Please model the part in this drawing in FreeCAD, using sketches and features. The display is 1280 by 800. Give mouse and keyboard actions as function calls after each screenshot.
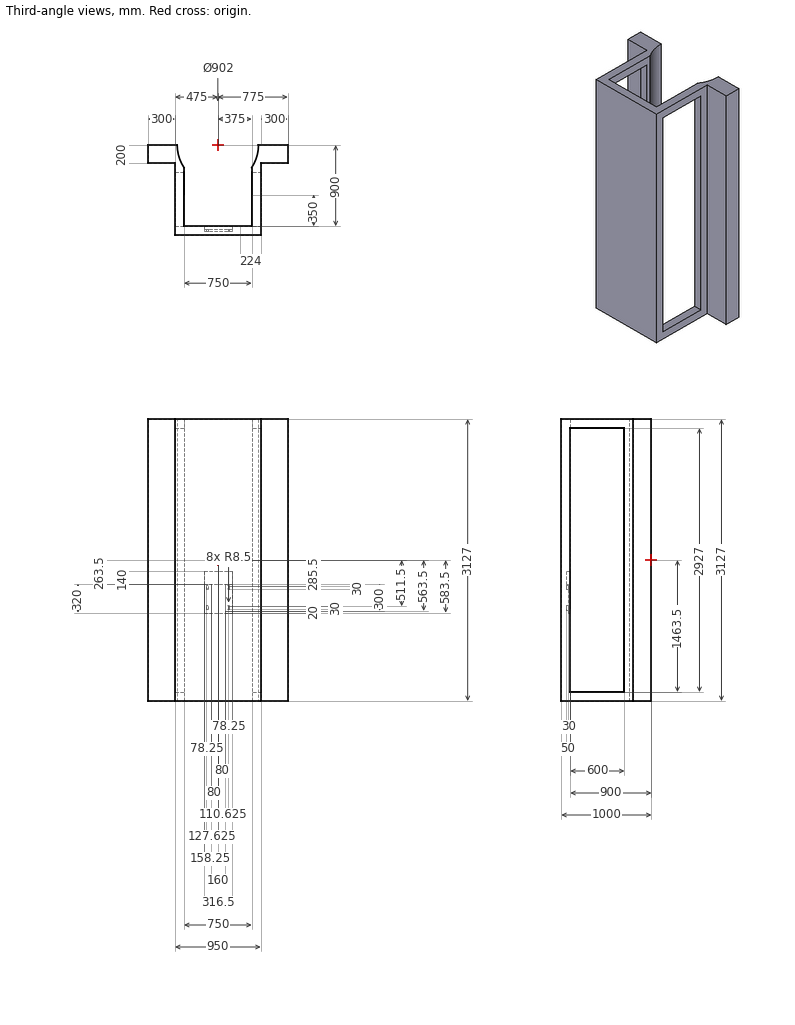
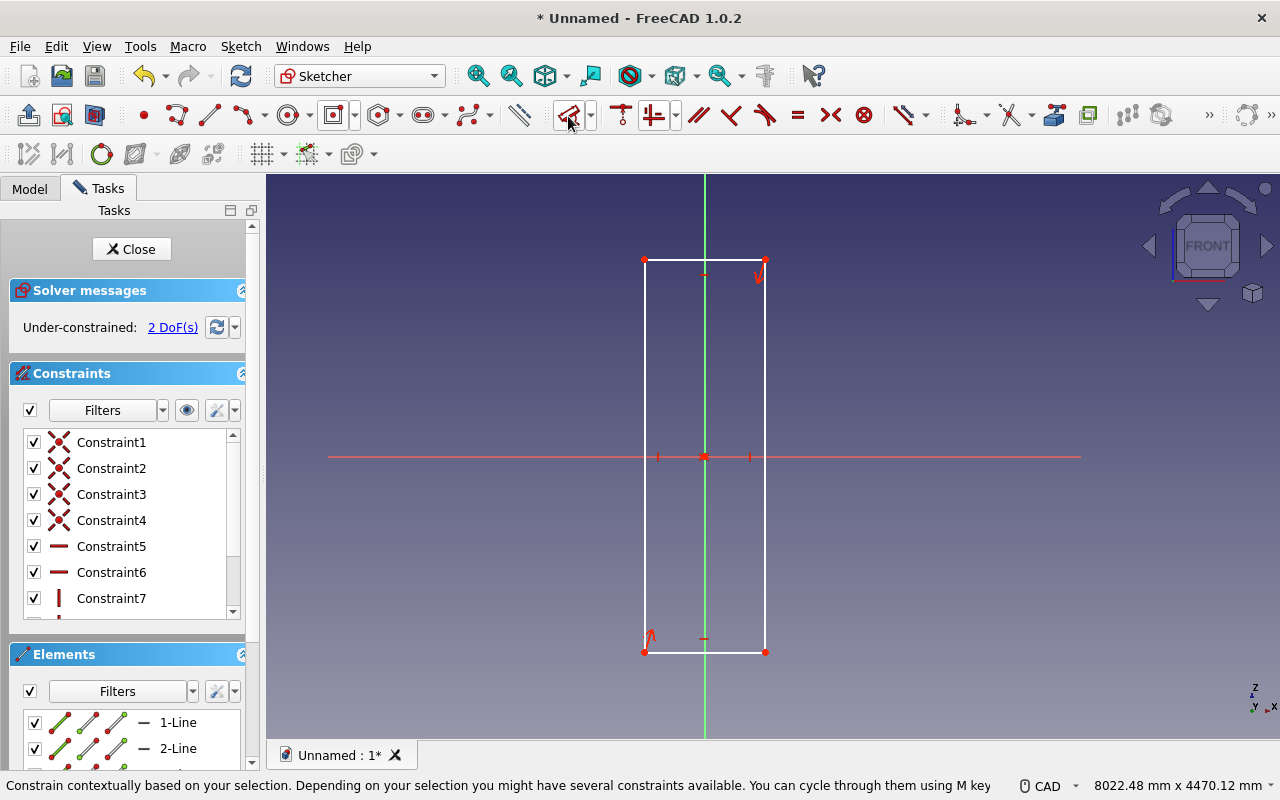
click(681, 653)
click(677, 687)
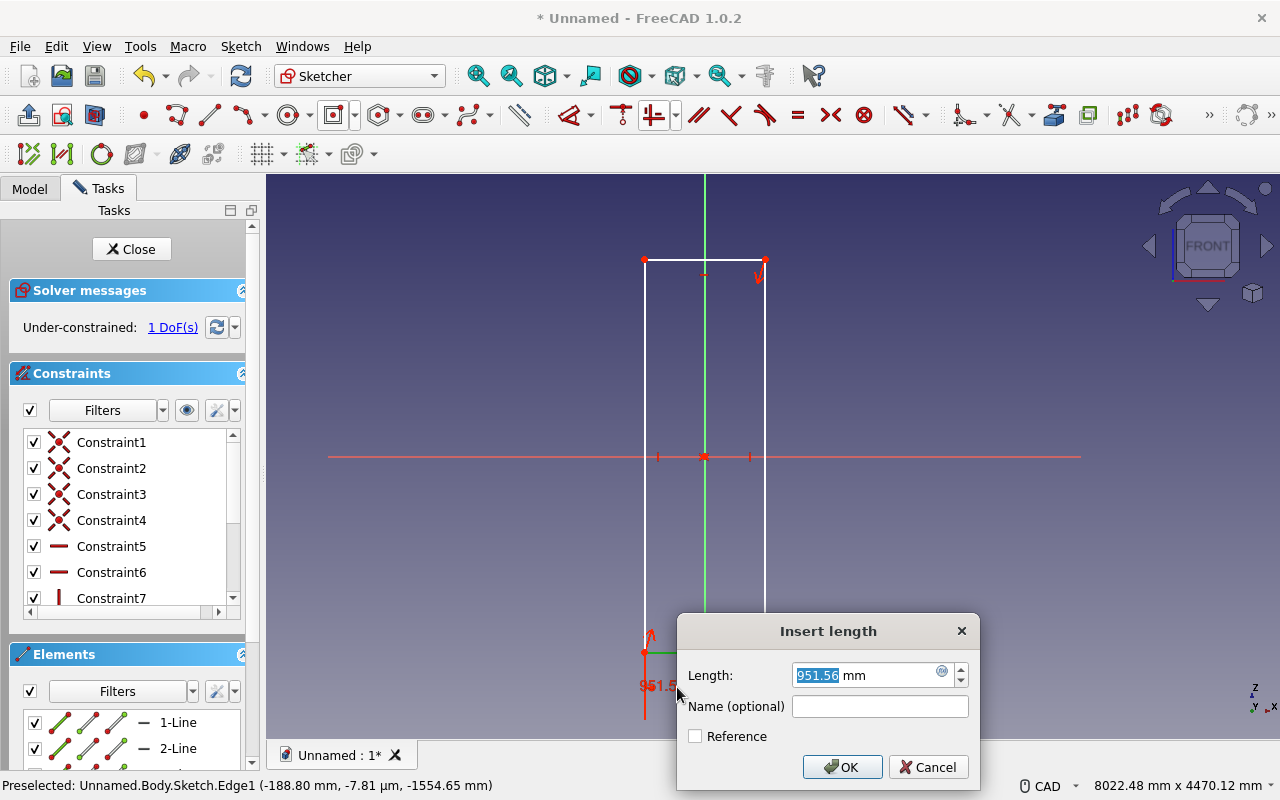
text(950)
key(Return)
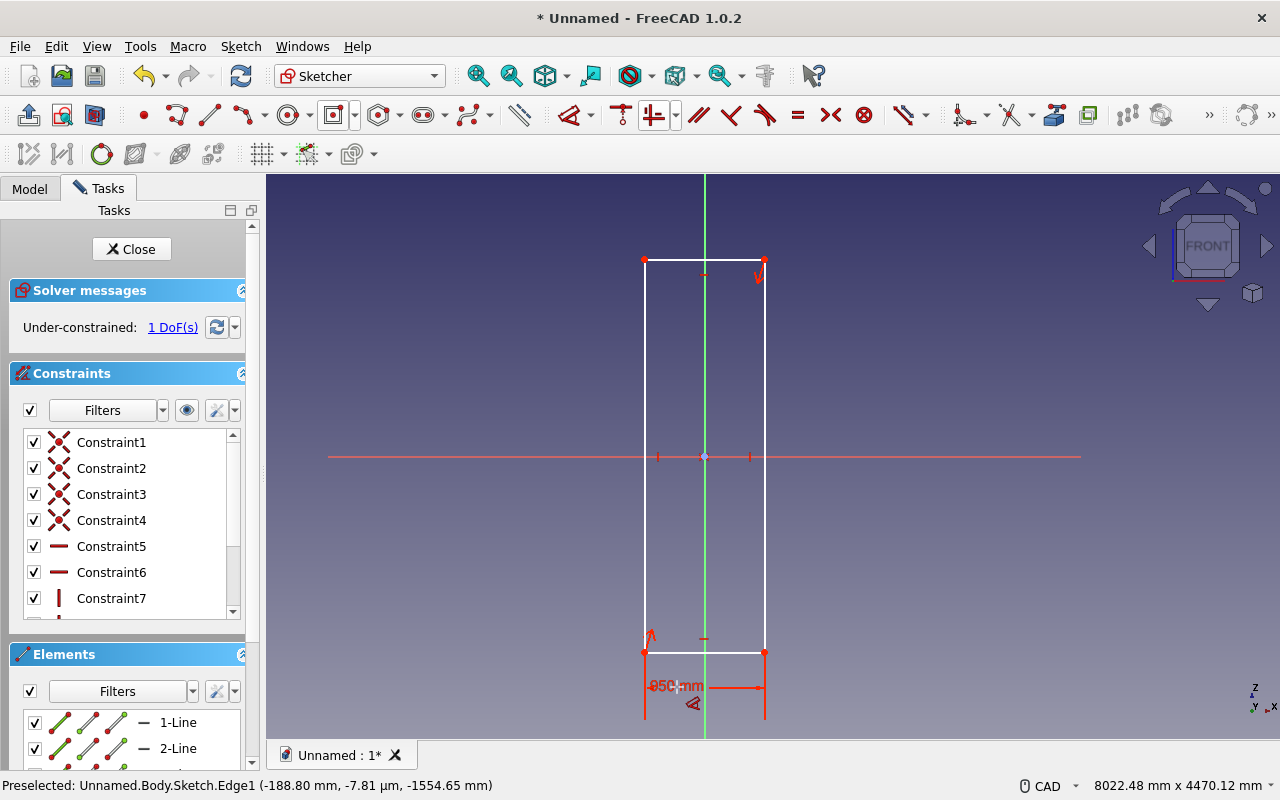
click(765, 535)
click(799, 366)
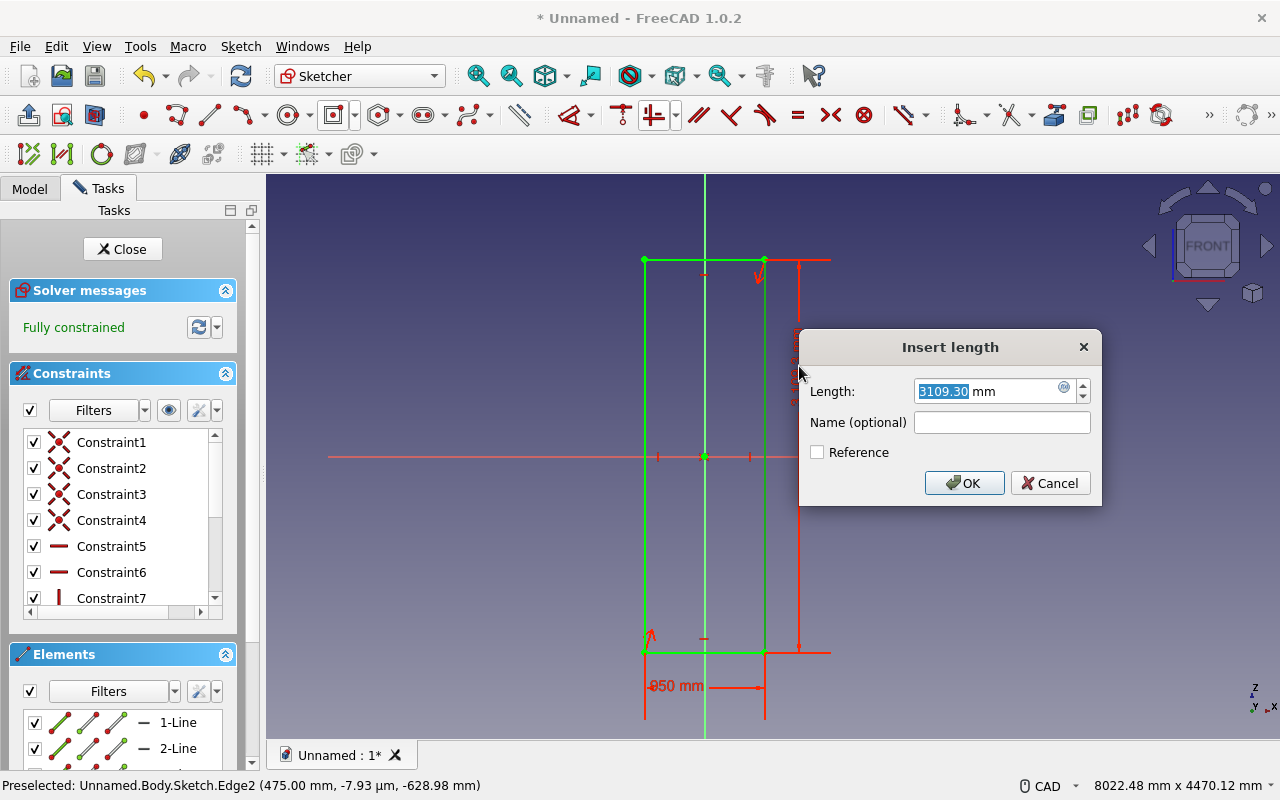
text(3127)
key(Return)
key(Escape)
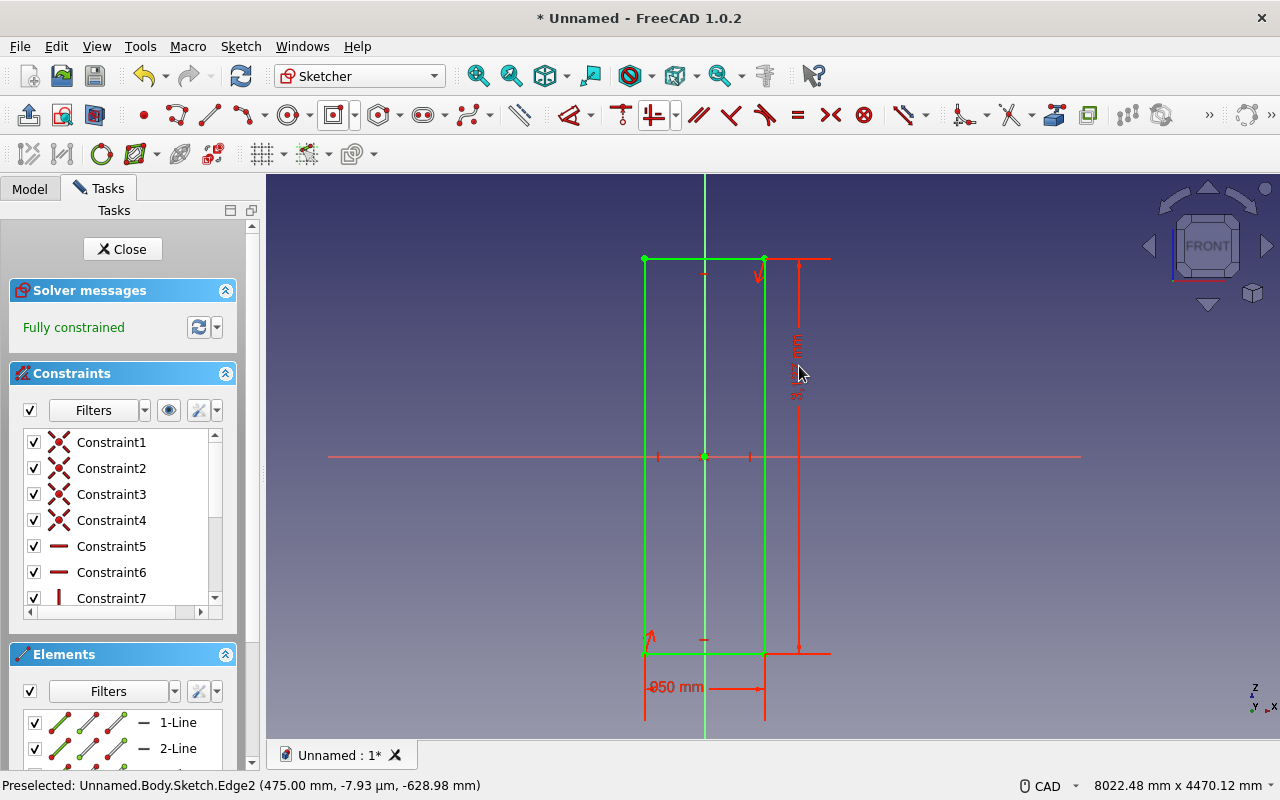
click(123, 249)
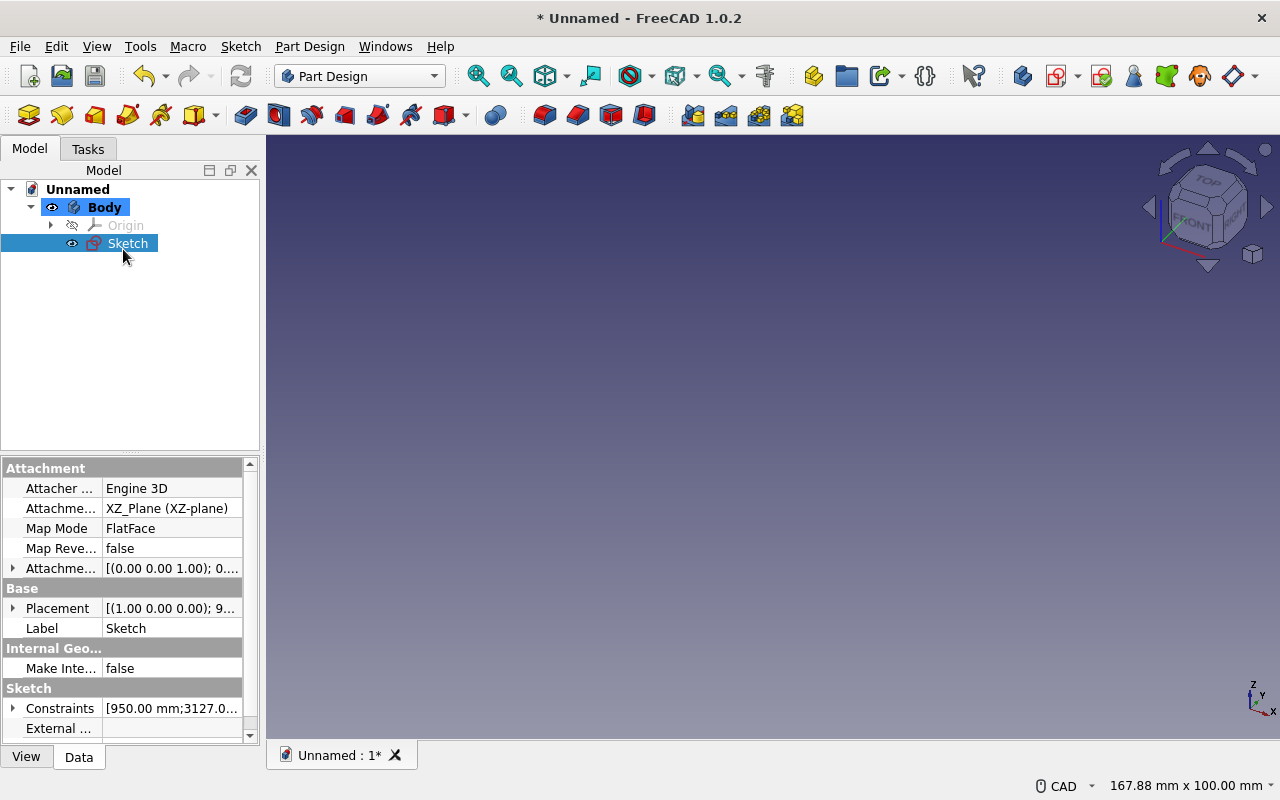
click(29, 116)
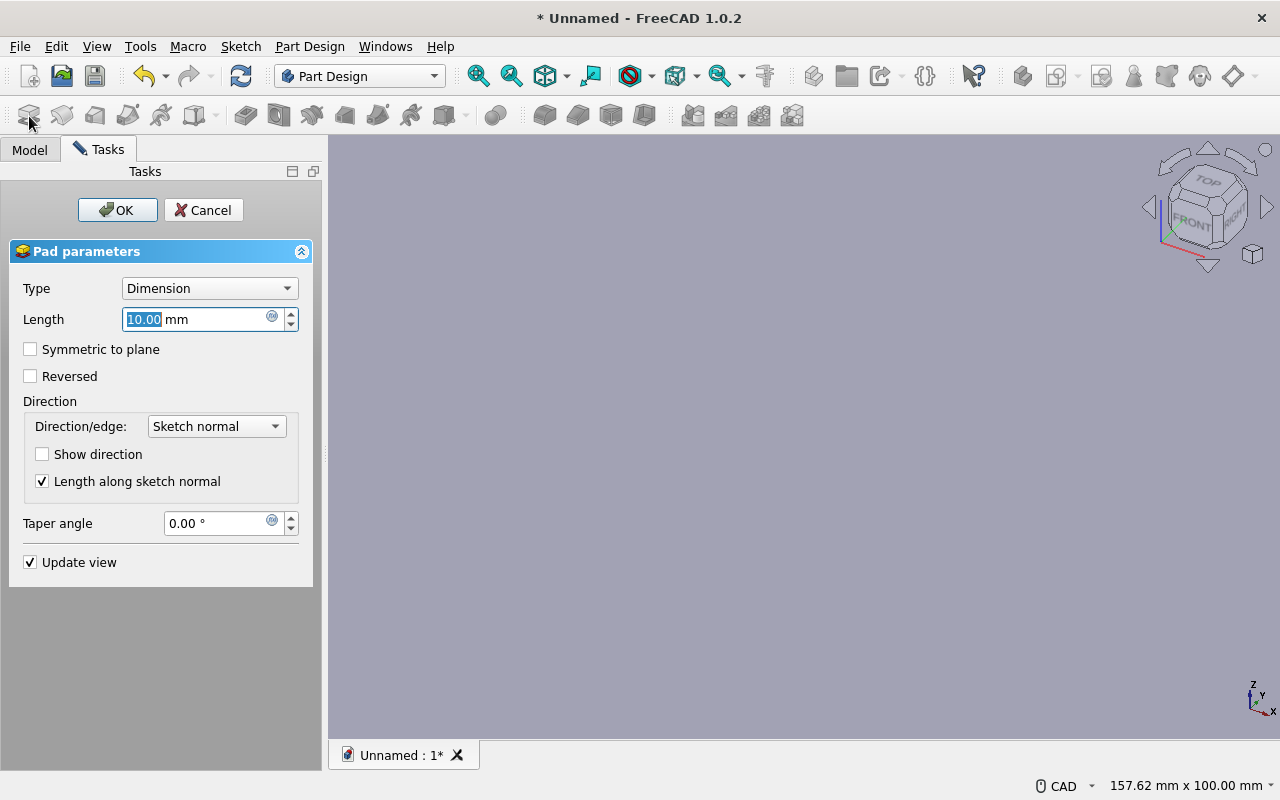
text(1000)
key(Tab)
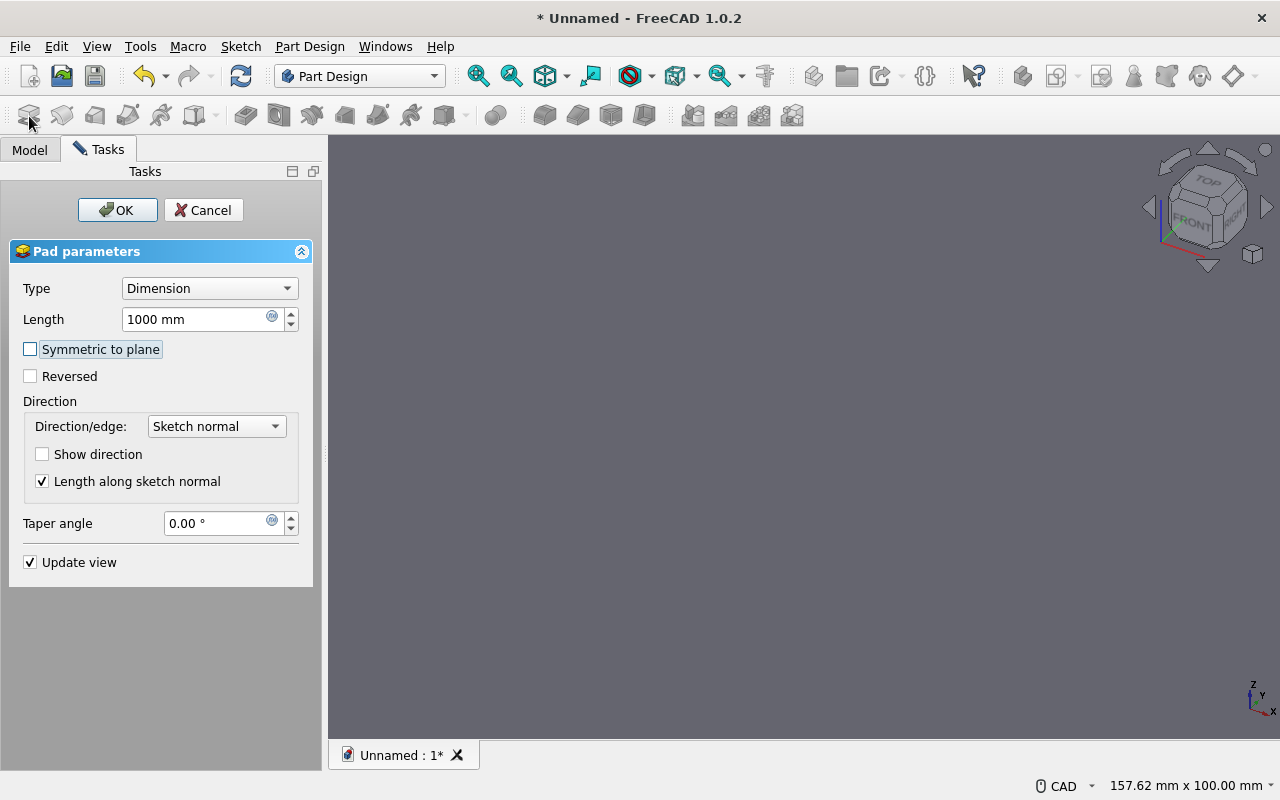
click(118, 210)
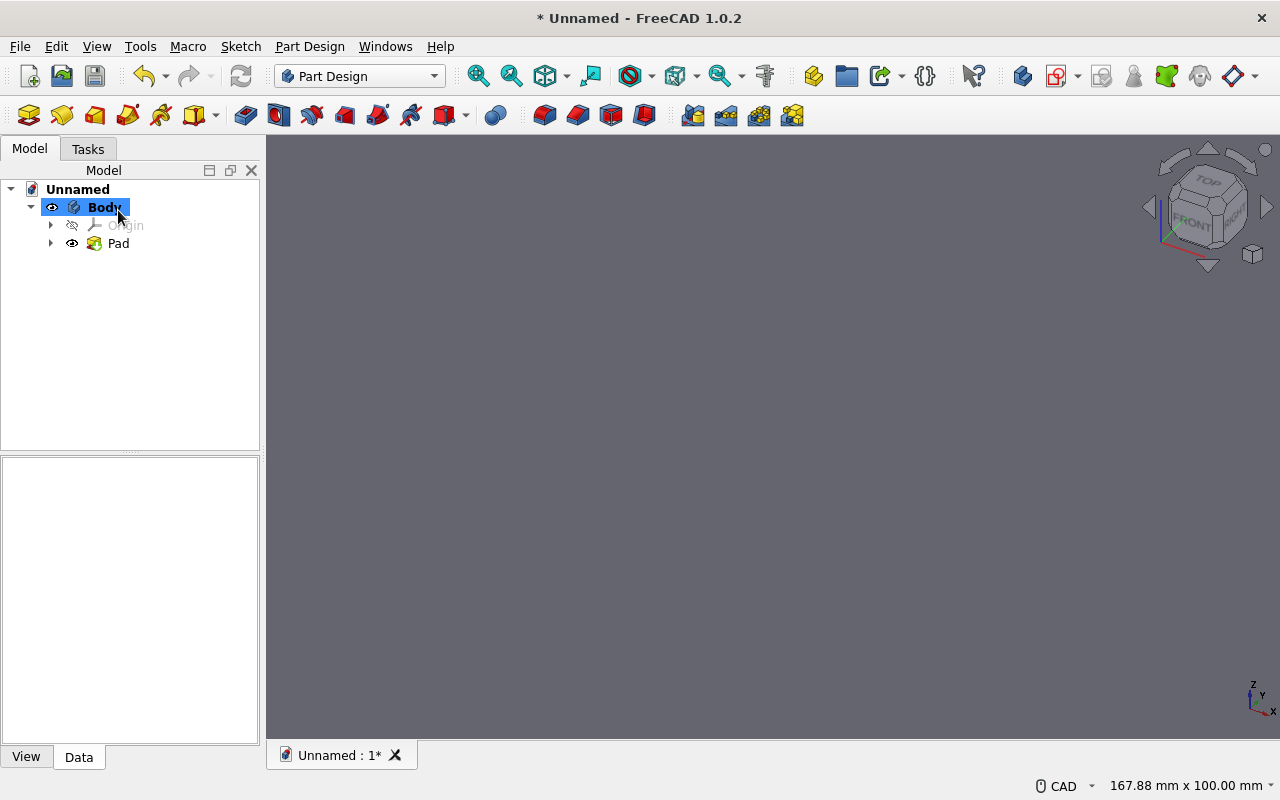
click(479, 76)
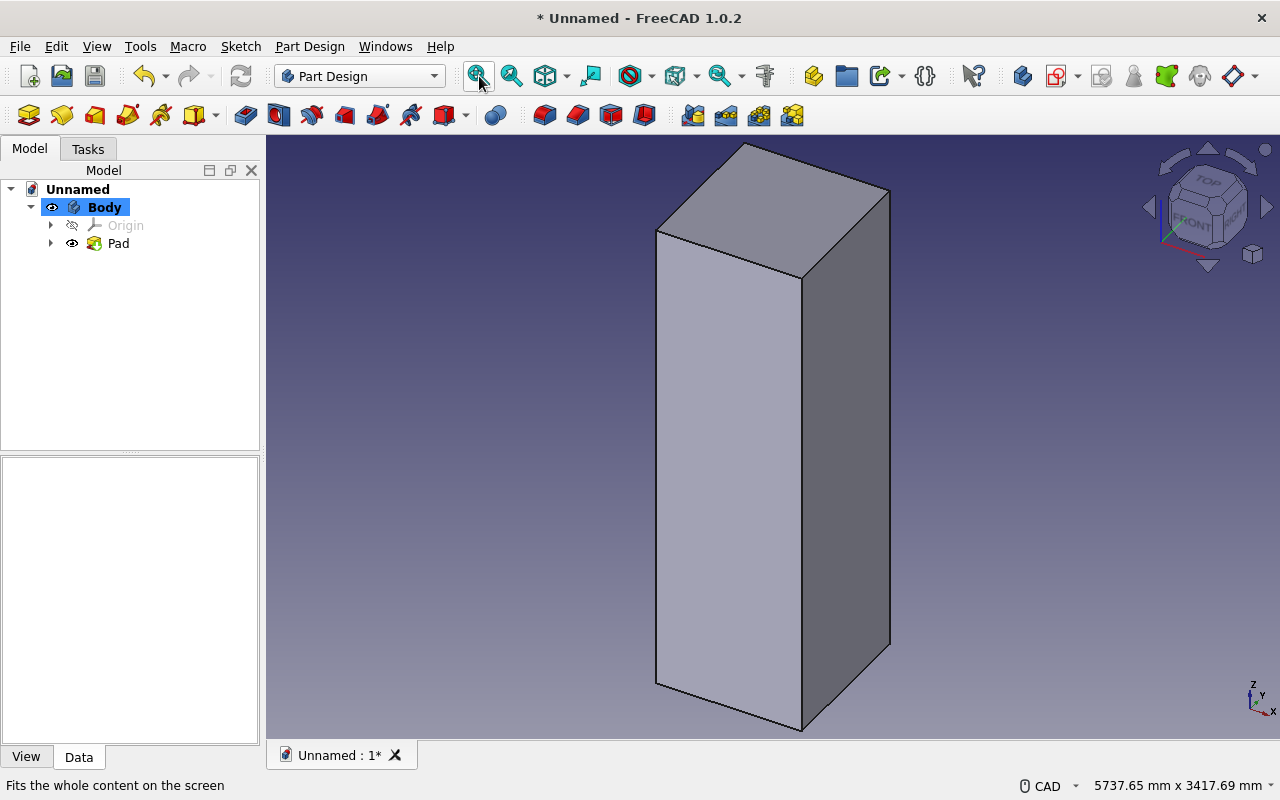
click(773, 210)